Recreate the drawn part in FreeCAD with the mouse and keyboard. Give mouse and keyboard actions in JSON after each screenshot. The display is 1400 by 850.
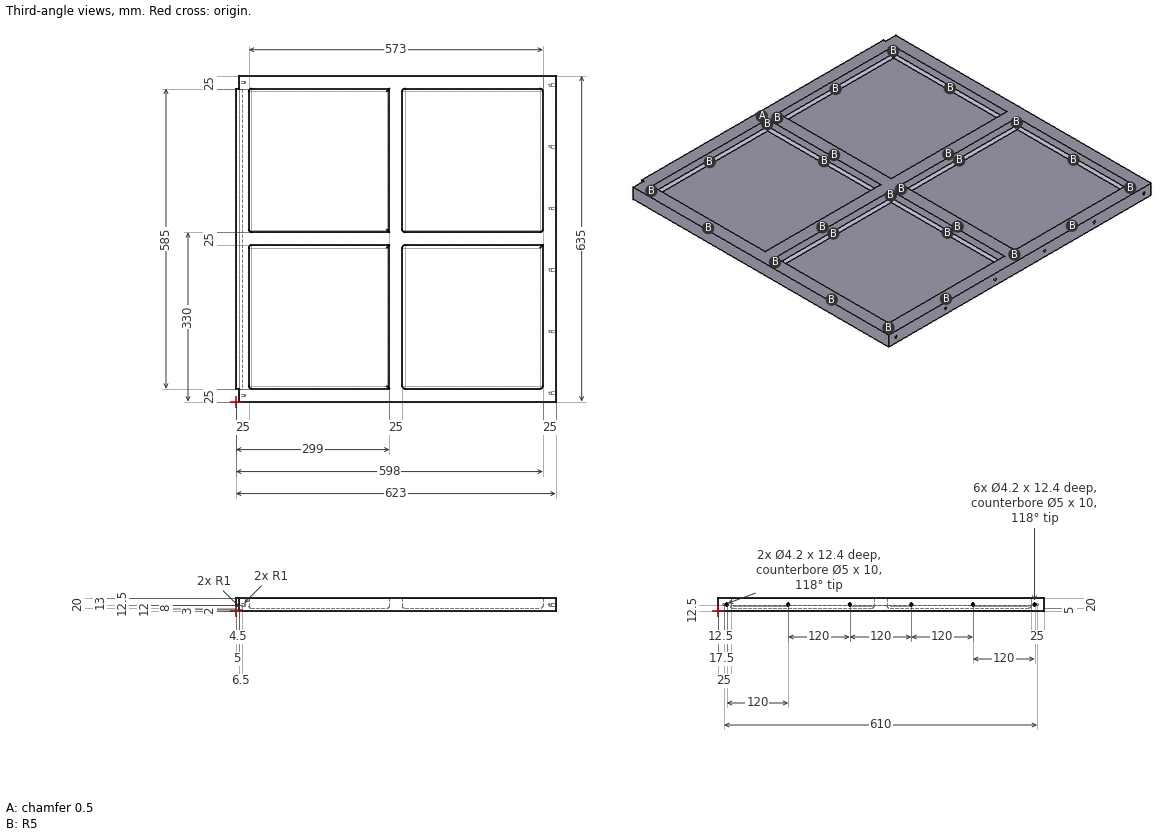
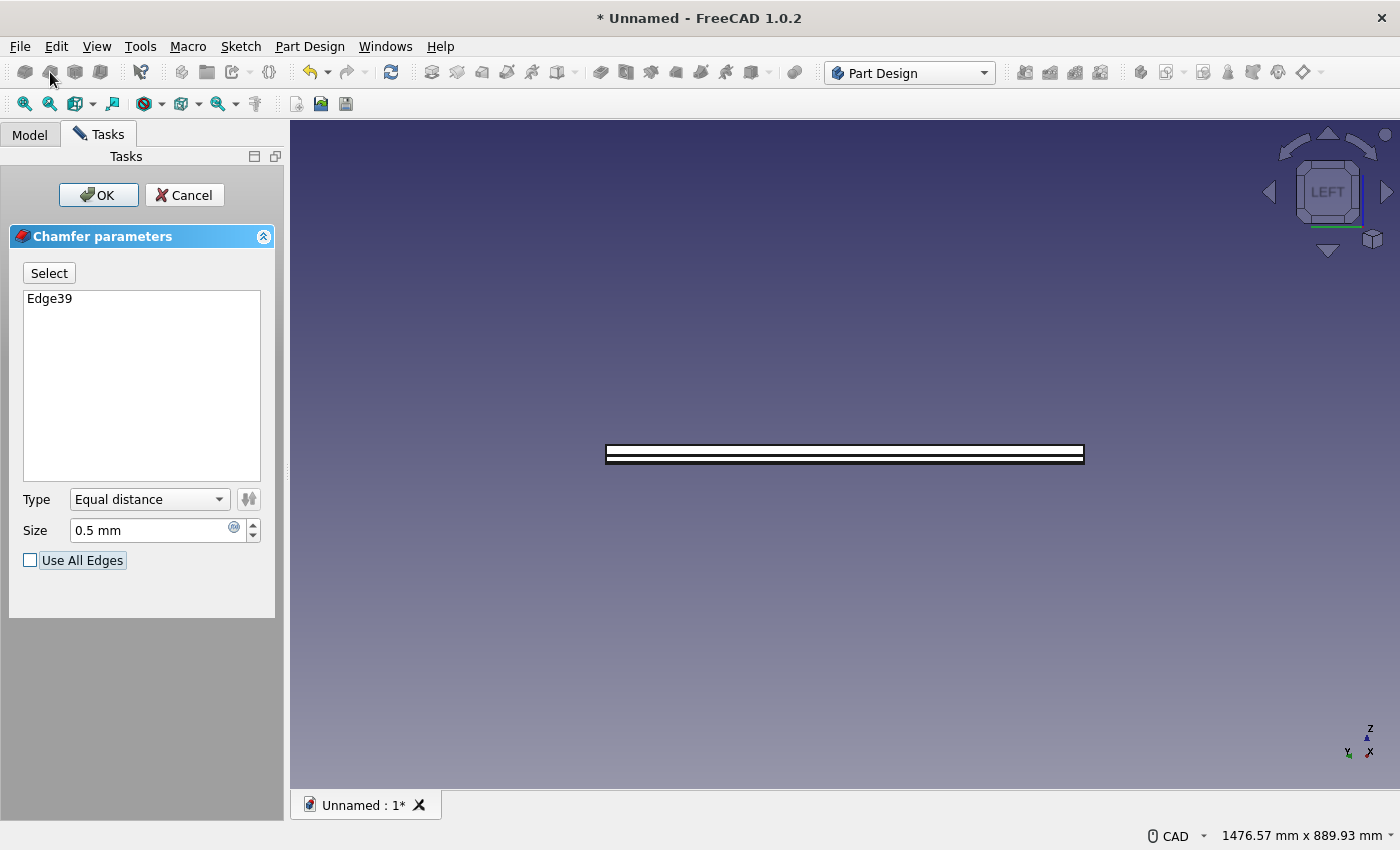
{"action": "left_click", "coordinate": [99, 195]}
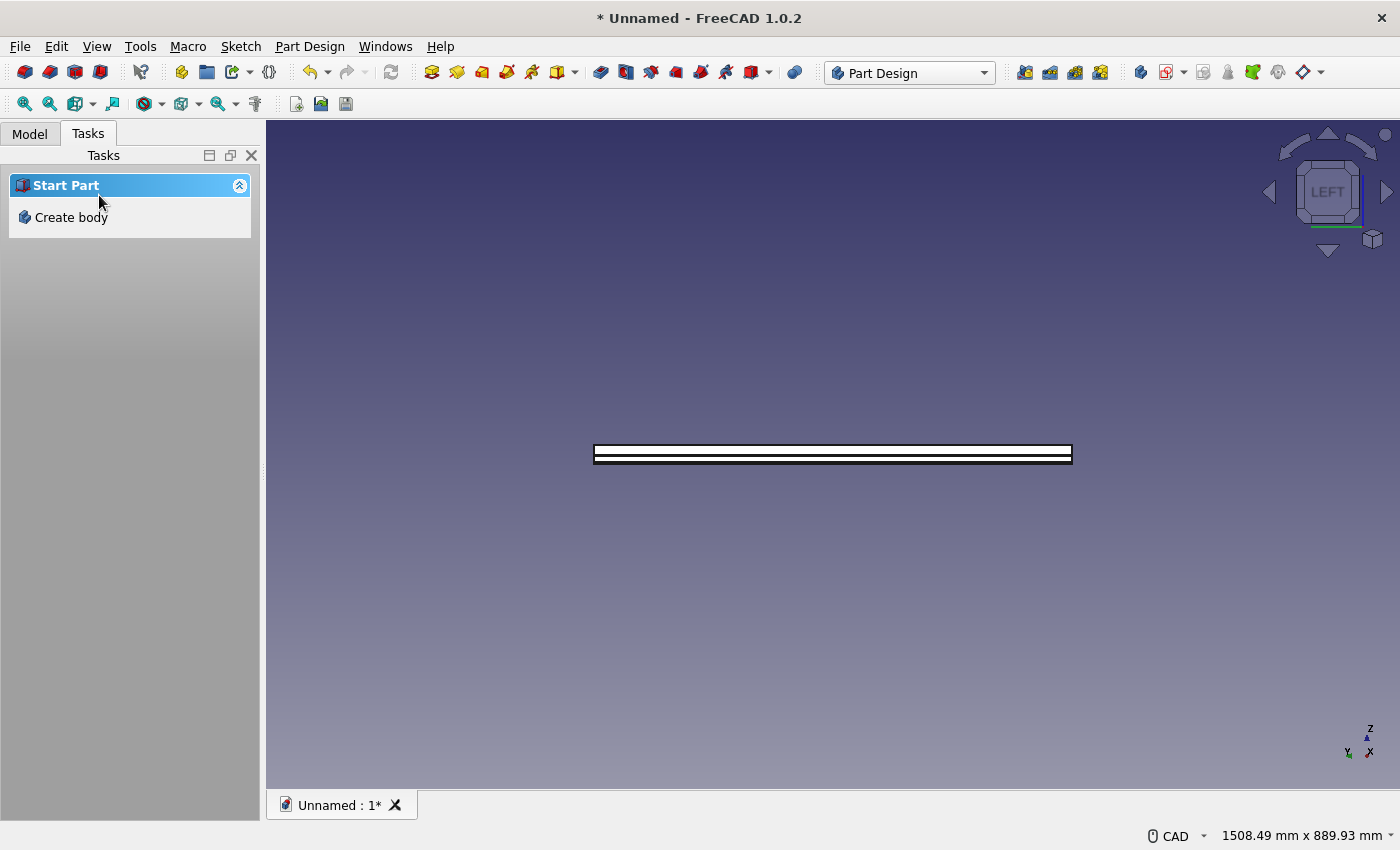
{"action": "left_click", "coordinate": [25, 104]}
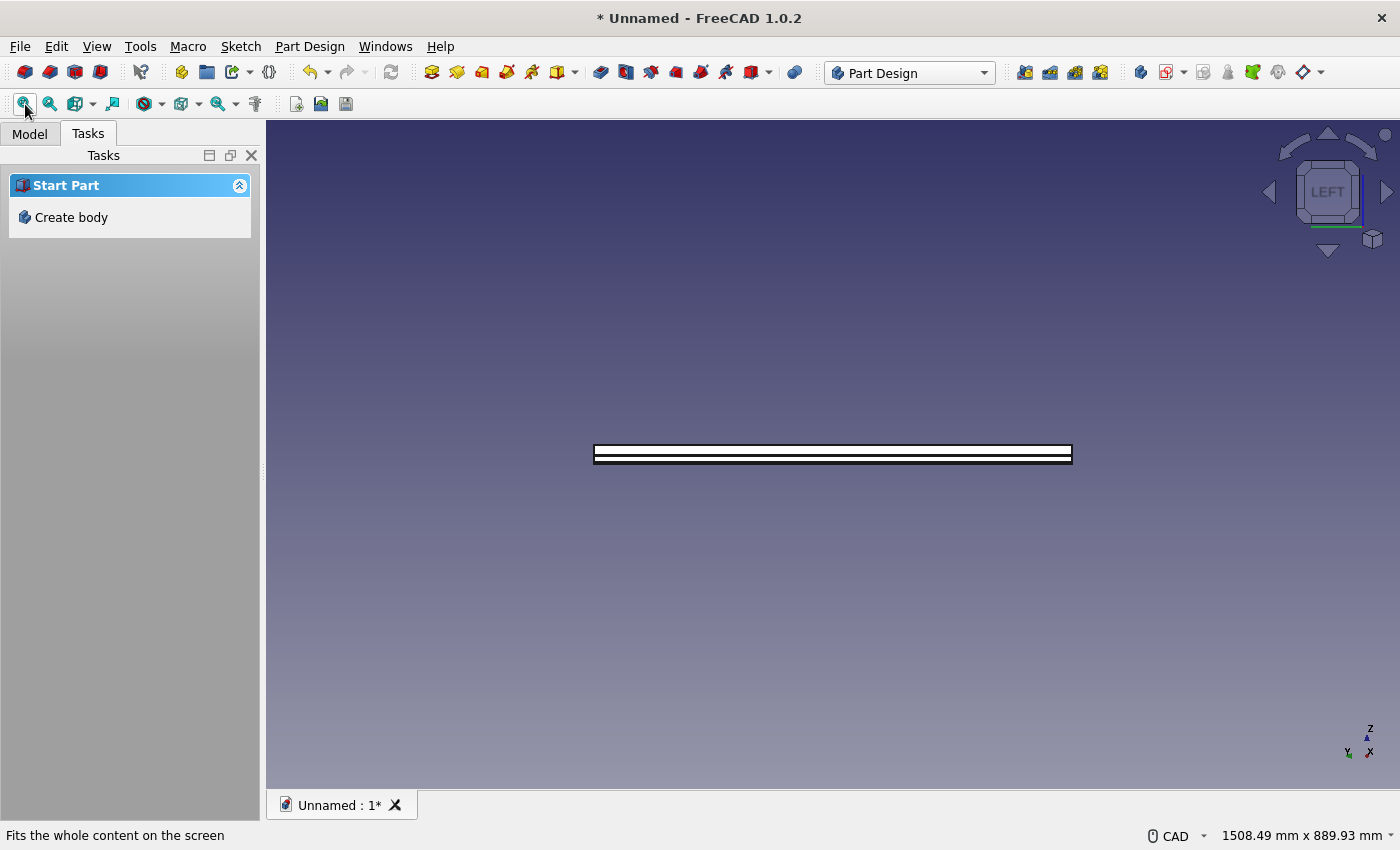
{"action": "key", "text": "0"}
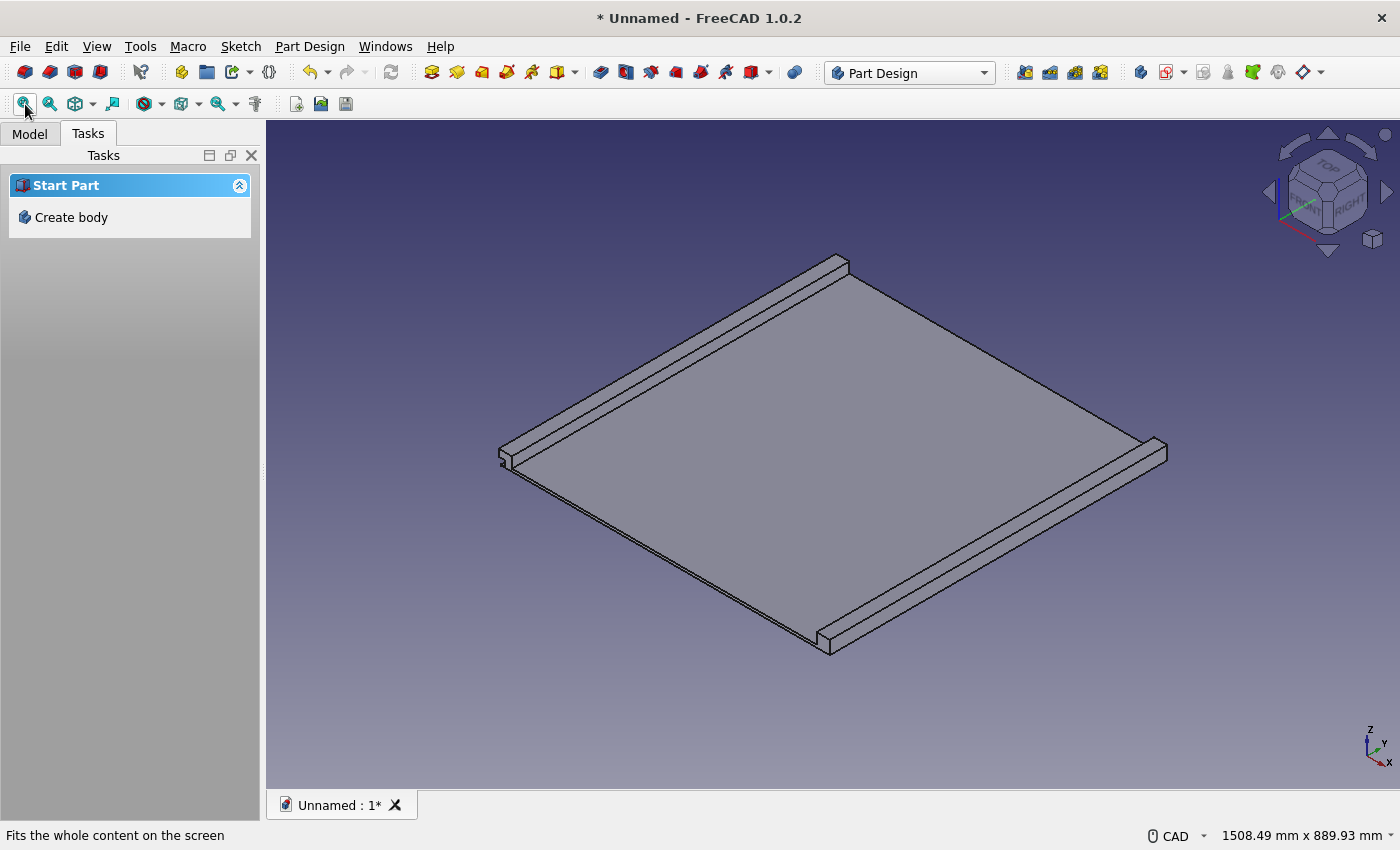
{"action": "left_click", "coordinate": [833, 458]}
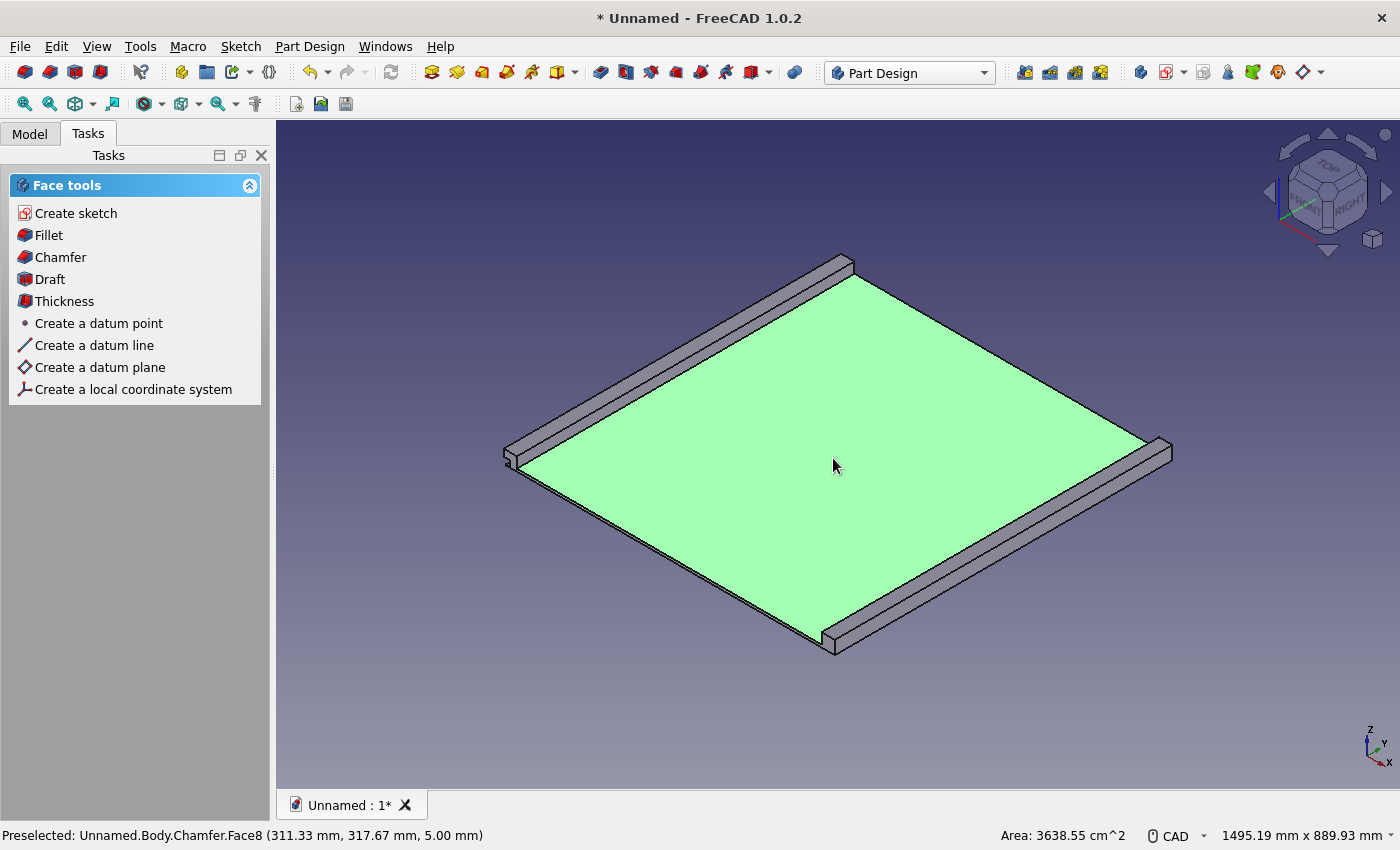
{"action": "left_click", "coordinate": [1166, 72]}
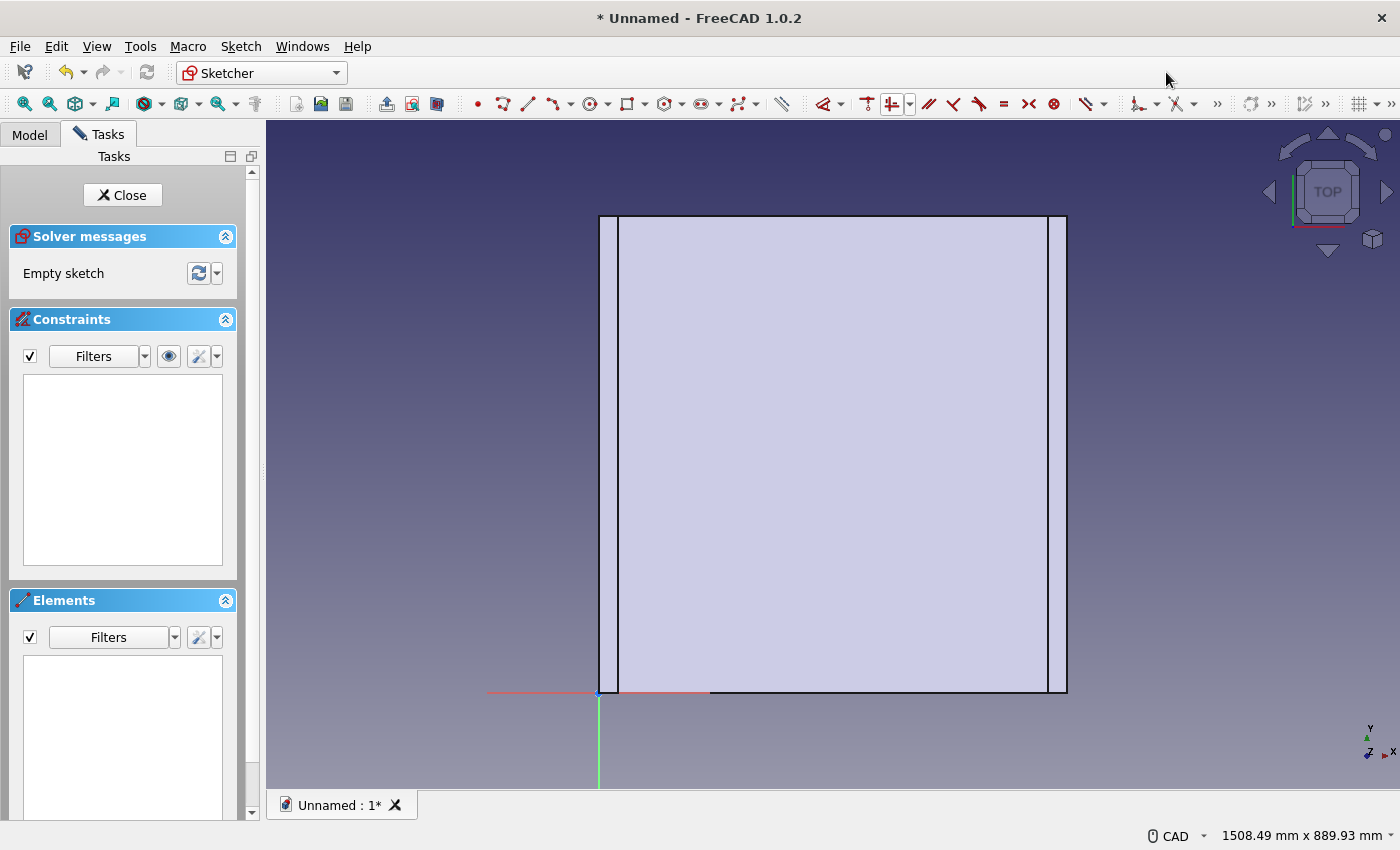
{"action": "left_click", "coordinate": [437, 104]}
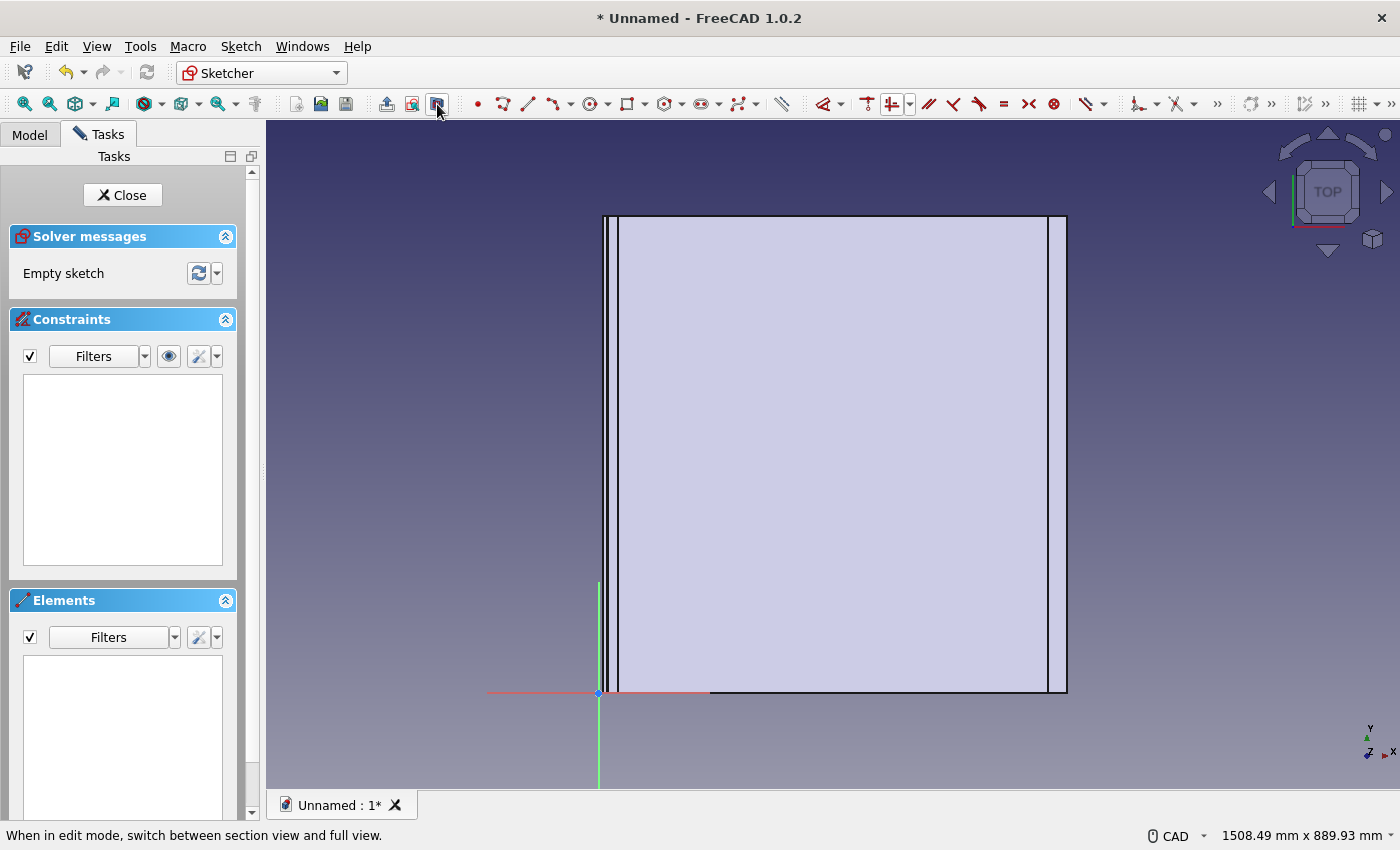
{"action": "left_click", "coordinate": [626, 104]}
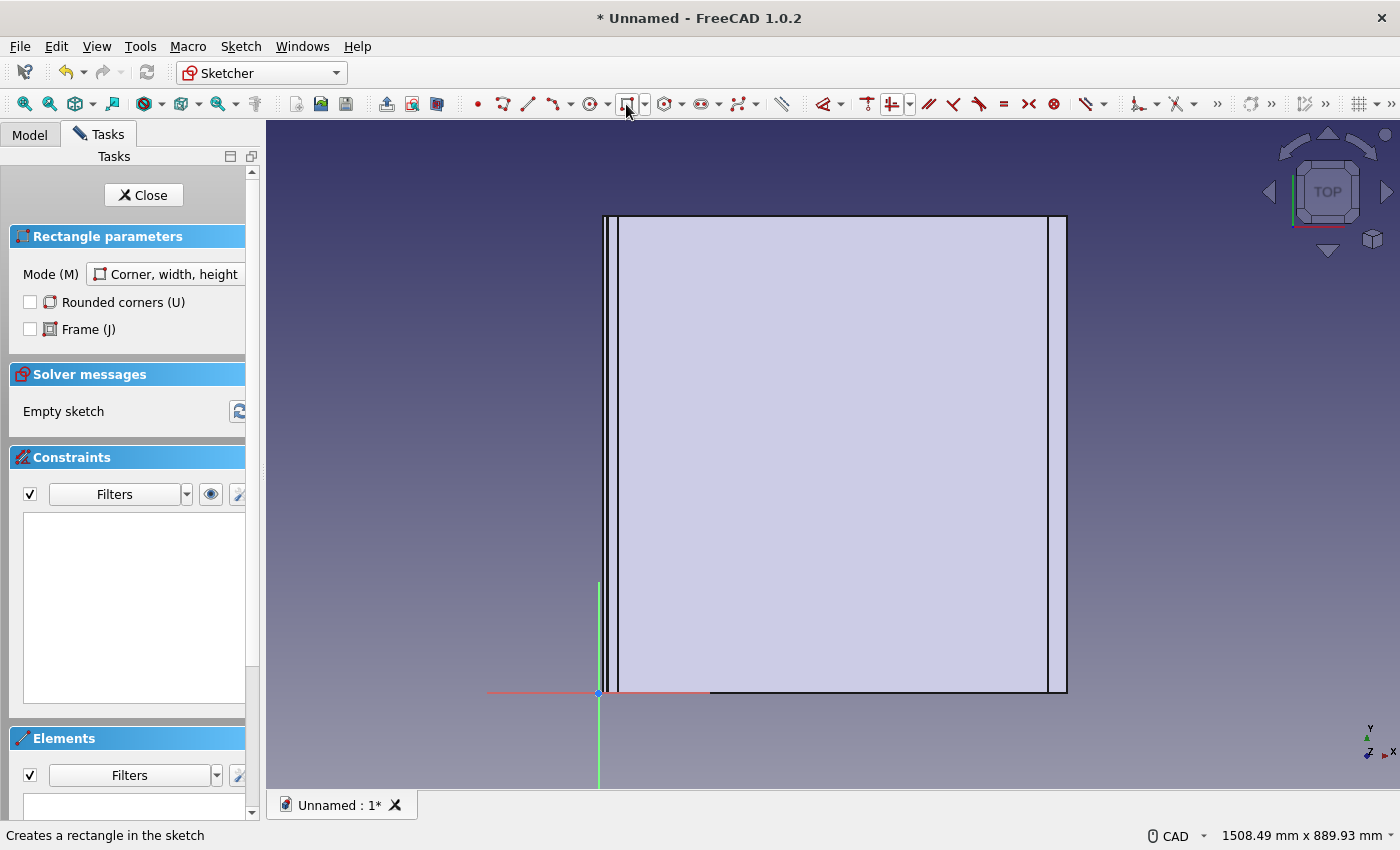
{"action": "left_click", "coordinate": [618, 216]}
{"action": "left_click", "coordinate": [1048, 235]}
{"action": "key", "text": "Escape"}